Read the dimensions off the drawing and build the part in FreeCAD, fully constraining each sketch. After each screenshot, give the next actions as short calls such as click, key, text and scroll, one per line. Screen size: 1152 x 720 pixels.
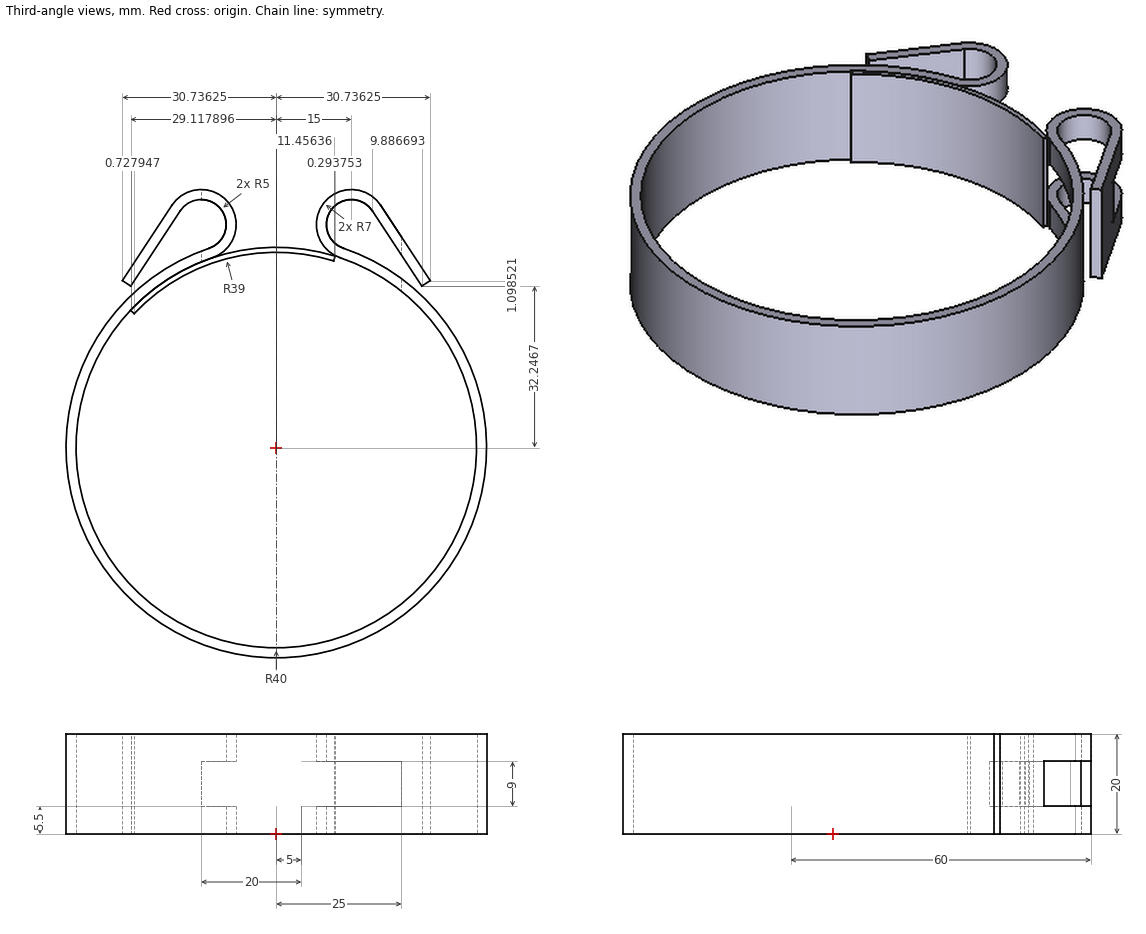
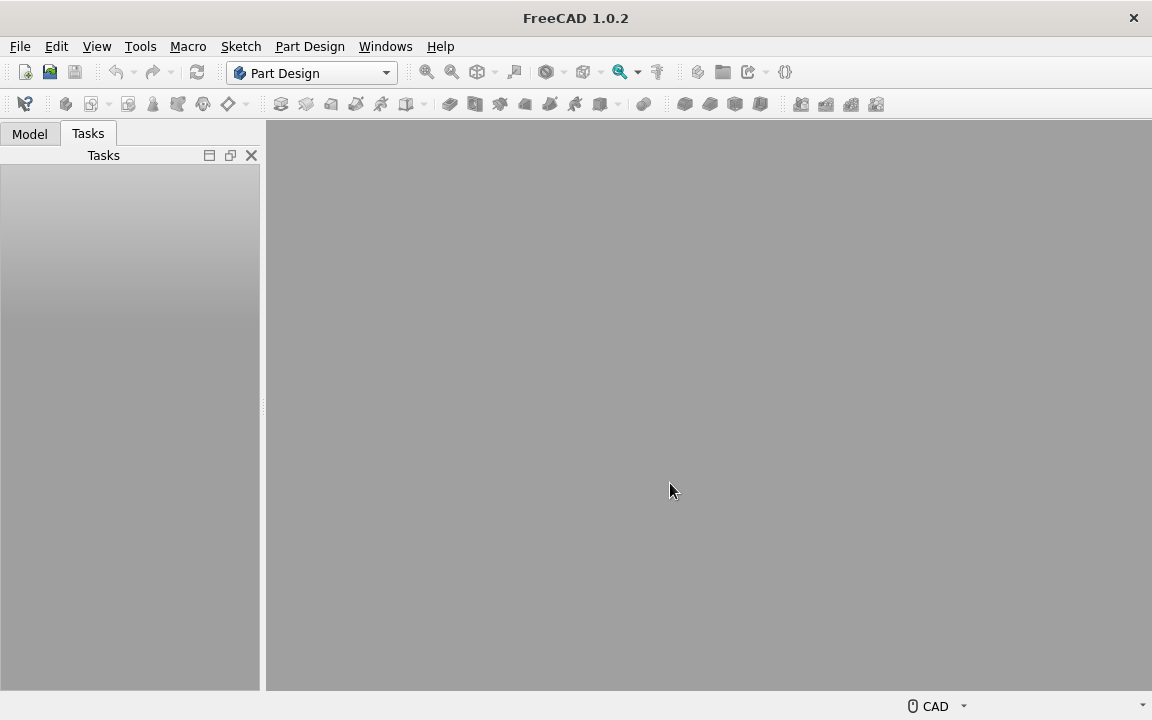
key(ctrl+n)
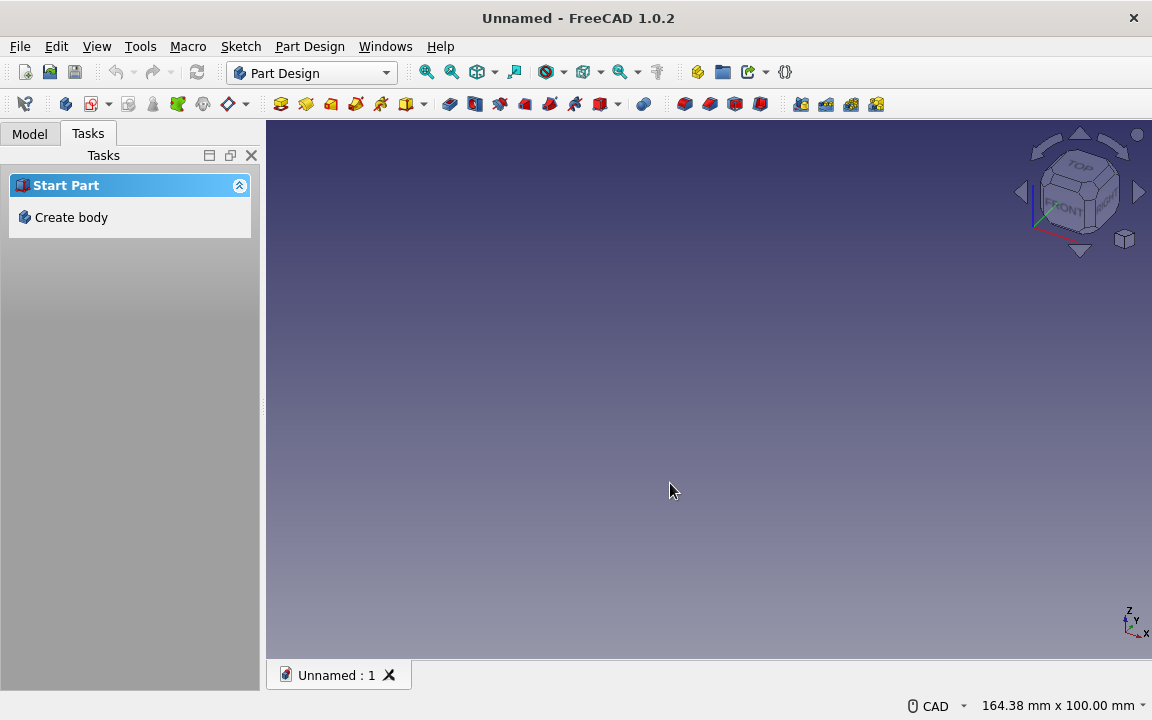
click(90, 104)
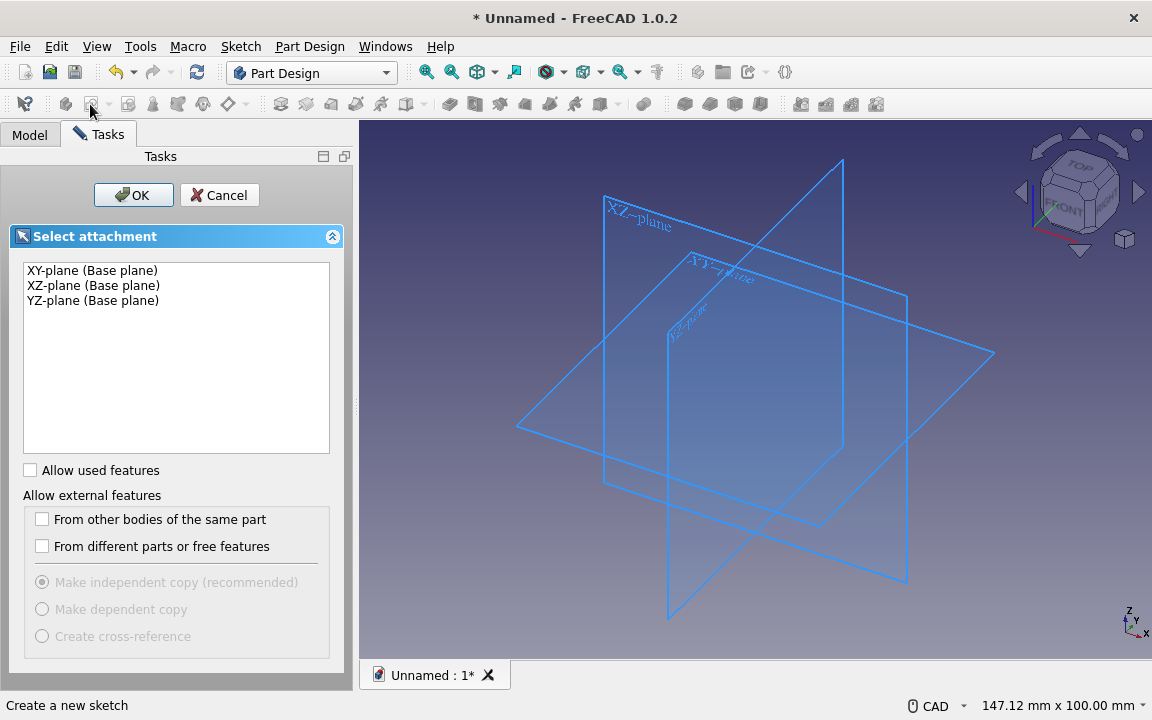
click(84, 270)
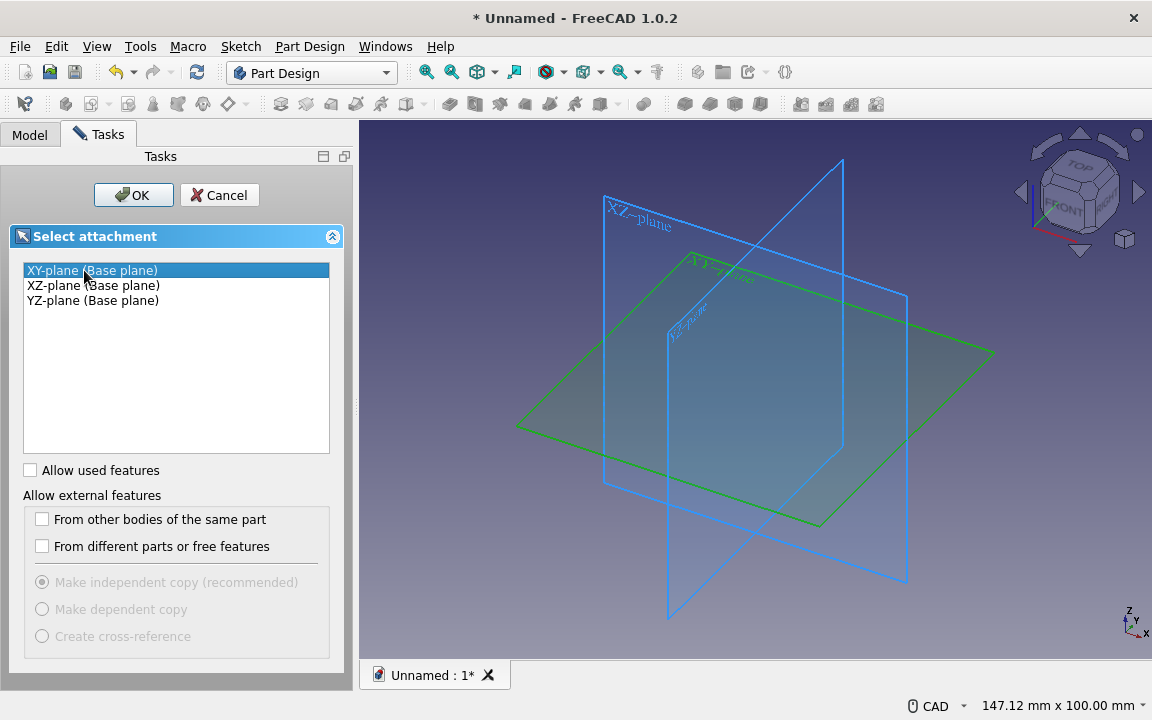
click(134, 195)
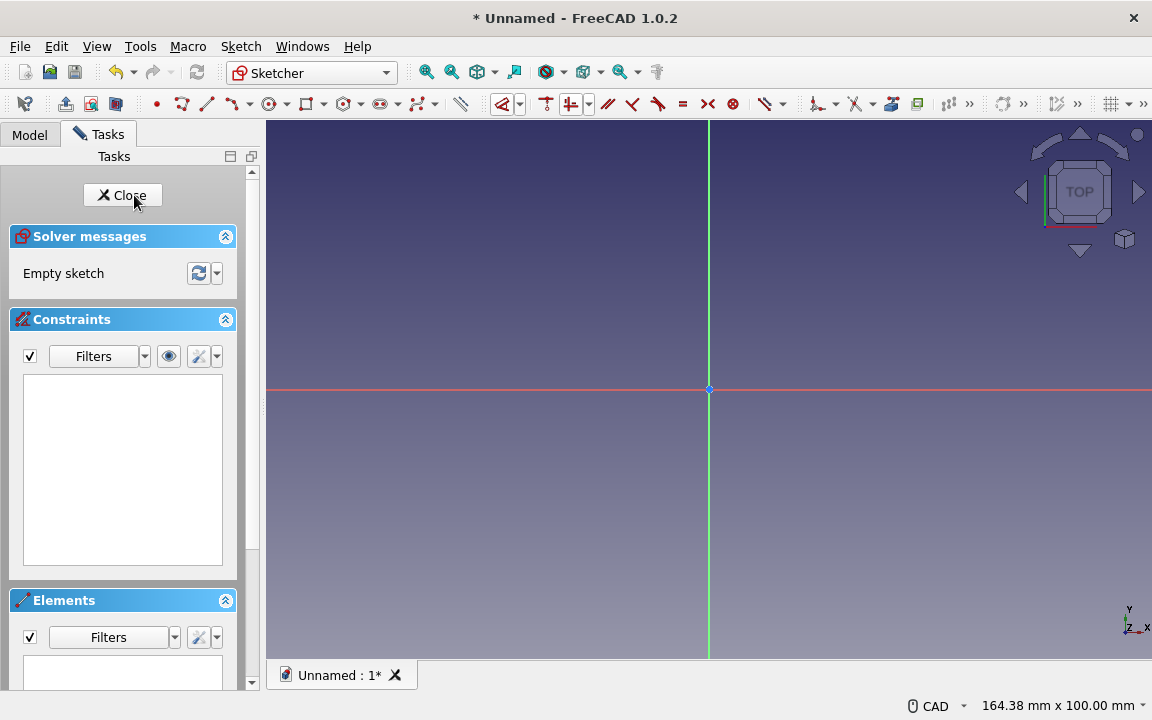
scroll(501, 427, down, 2)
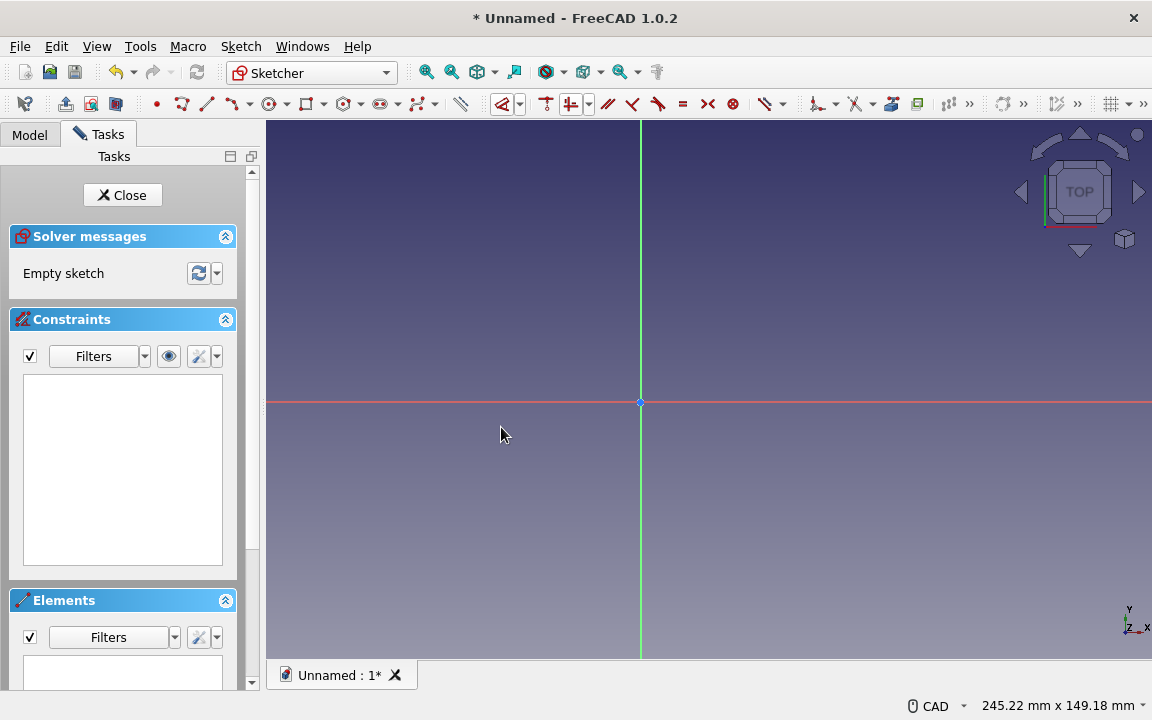
key(g)
key(m)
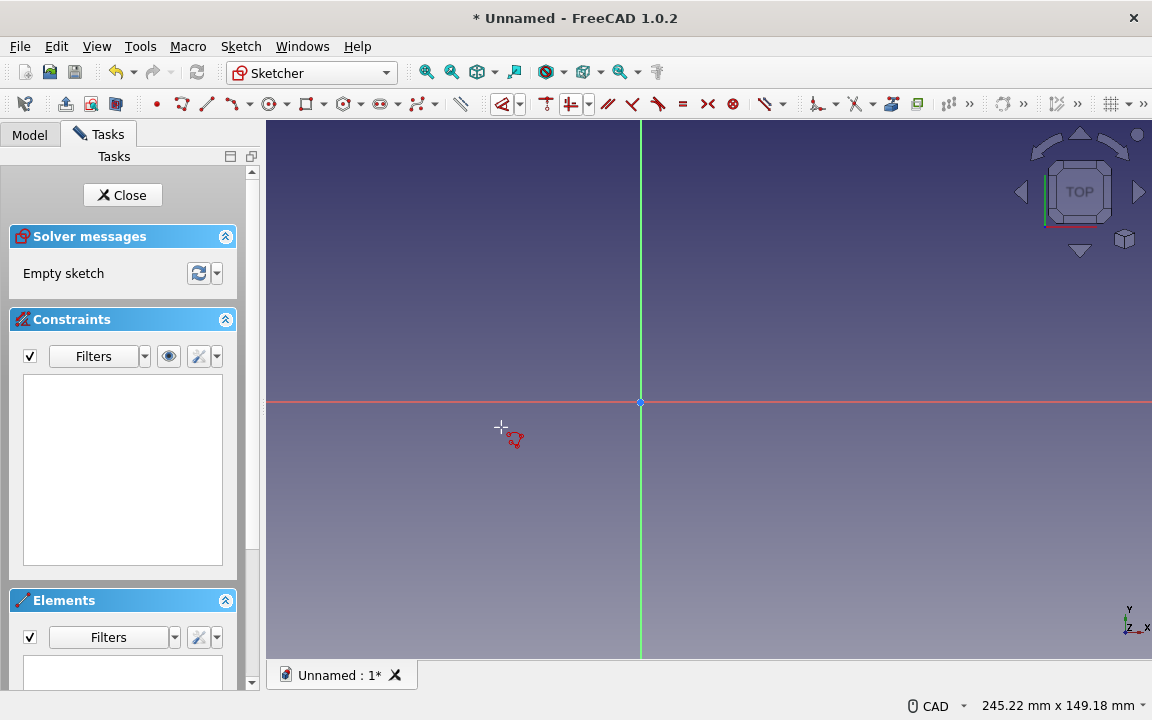
click(710, 231)
click(746, 286)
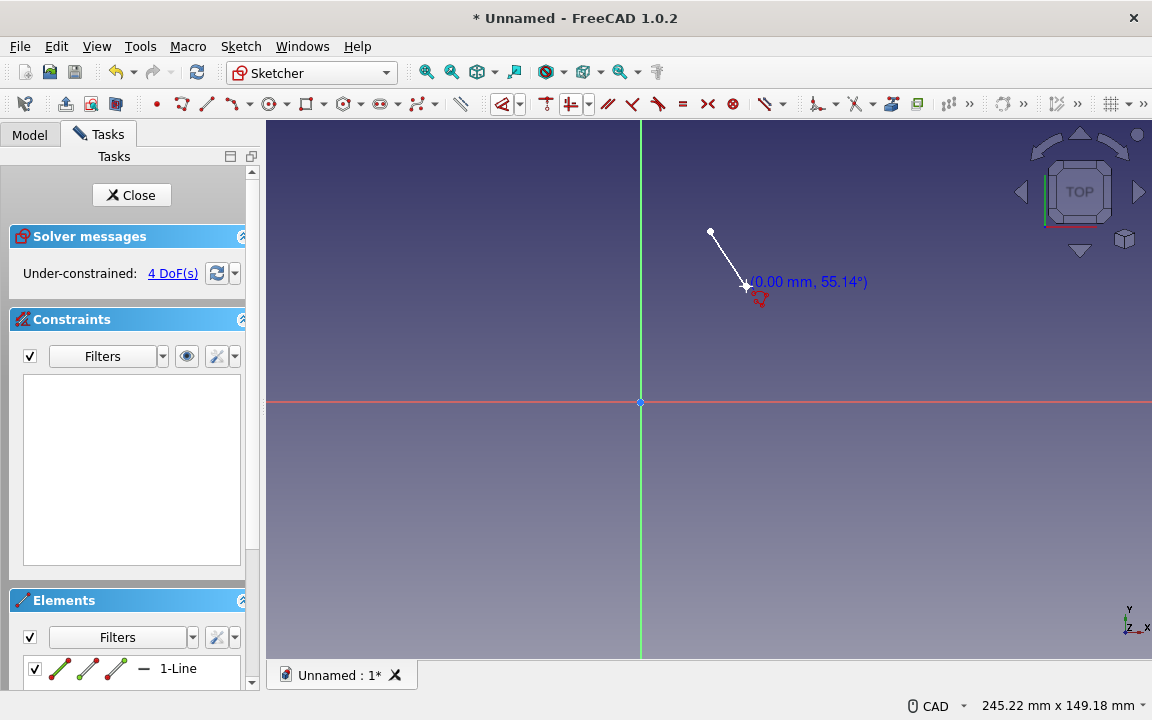
scroll(752, 282, up, 4)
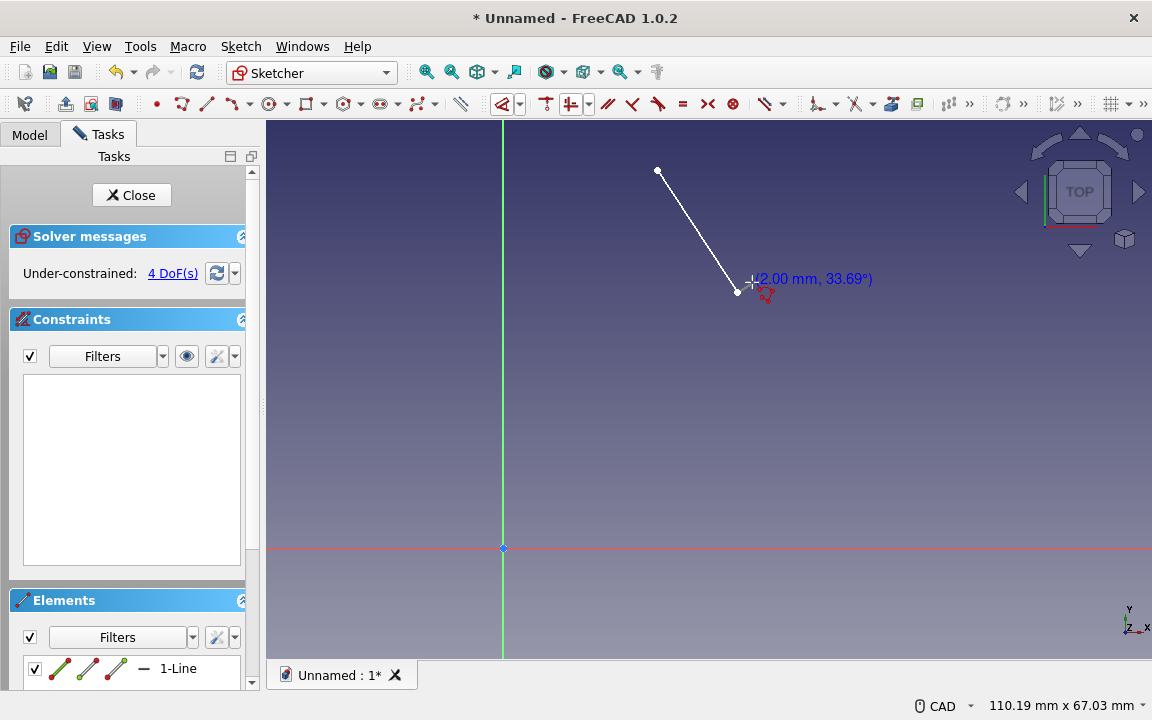
click(750, 281)
click(671, 160)
right_click(671, 160)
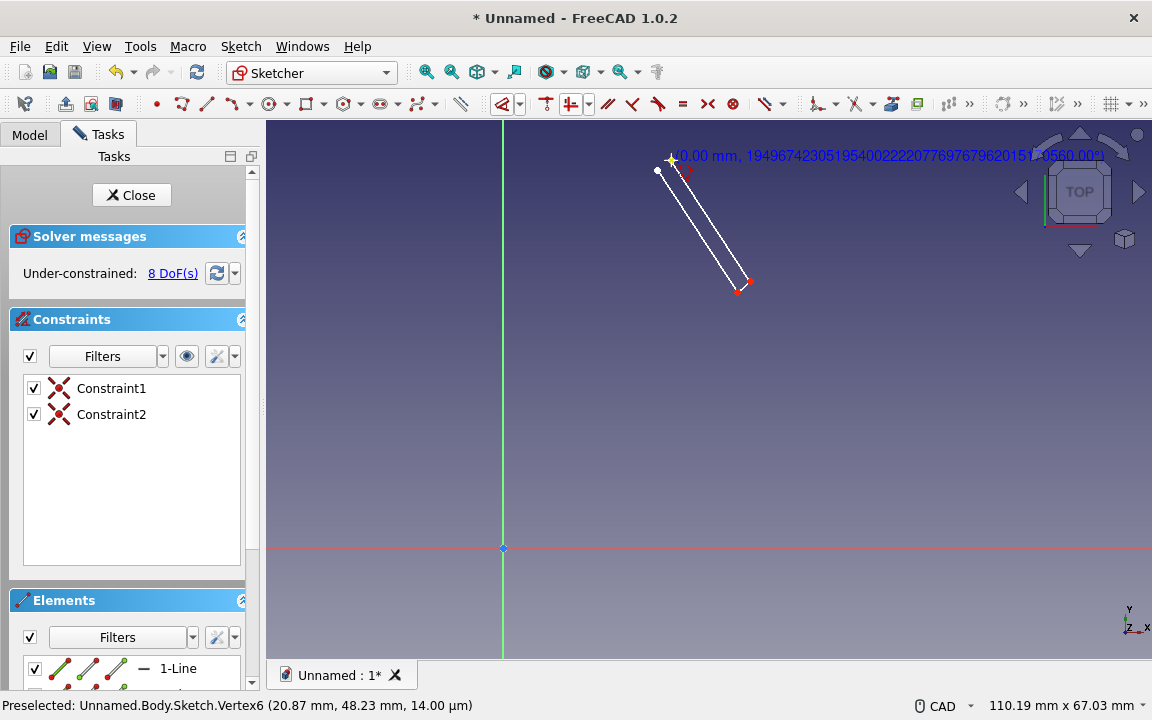
click(336, 160)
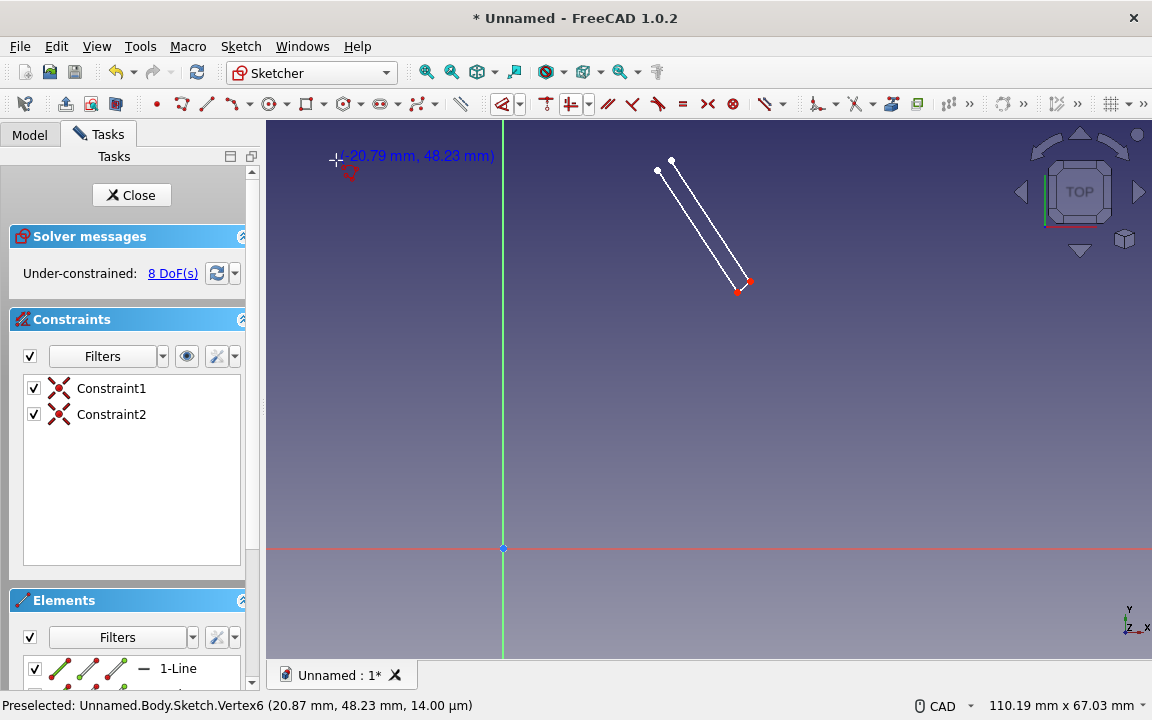
scroll(753, 282, down, 4)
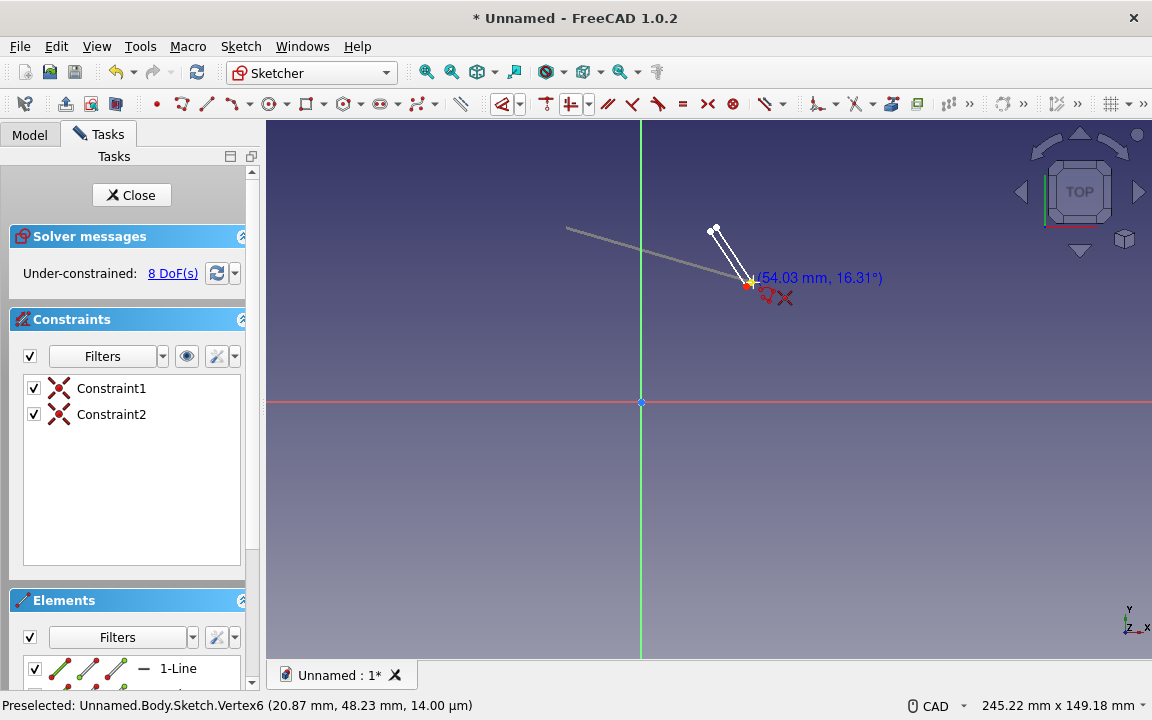
click(530, 282)